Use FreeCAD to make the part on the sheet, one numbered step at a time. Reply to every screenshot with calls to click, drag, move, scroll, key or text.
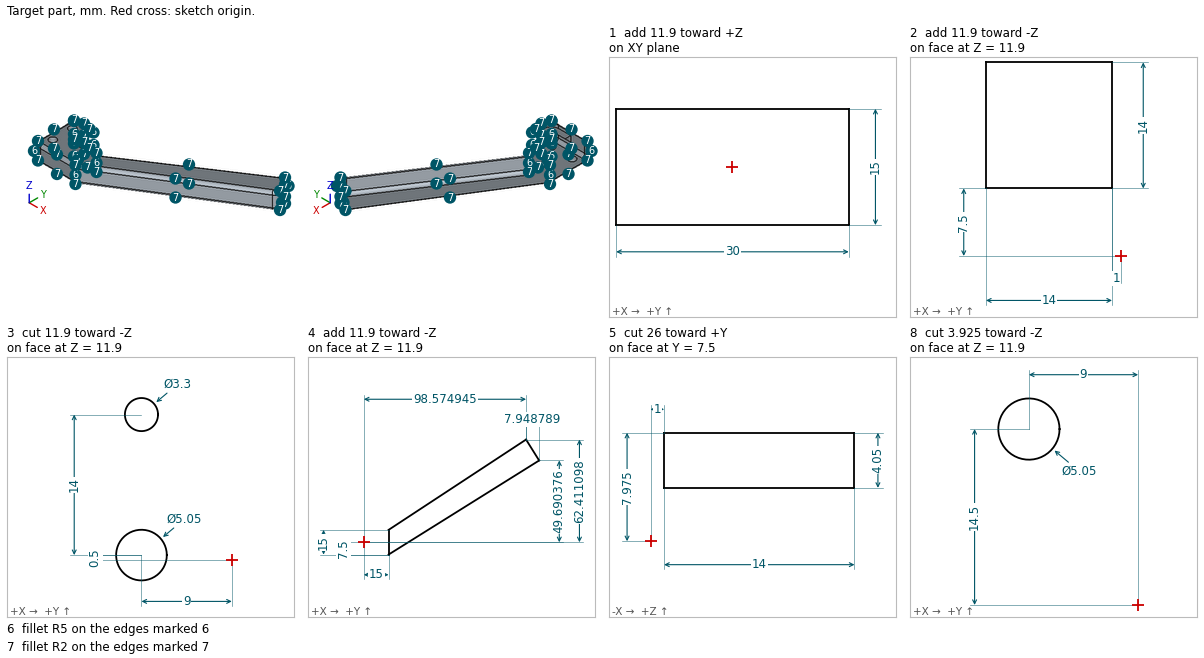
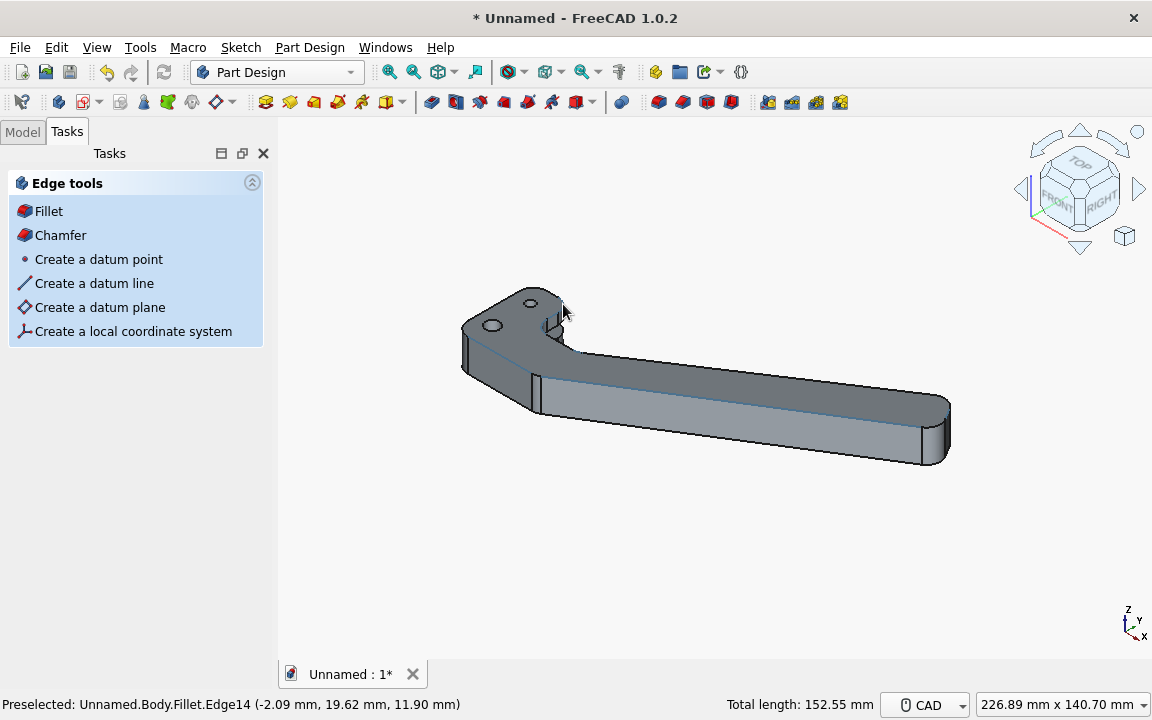
click(462, 328, ctrl)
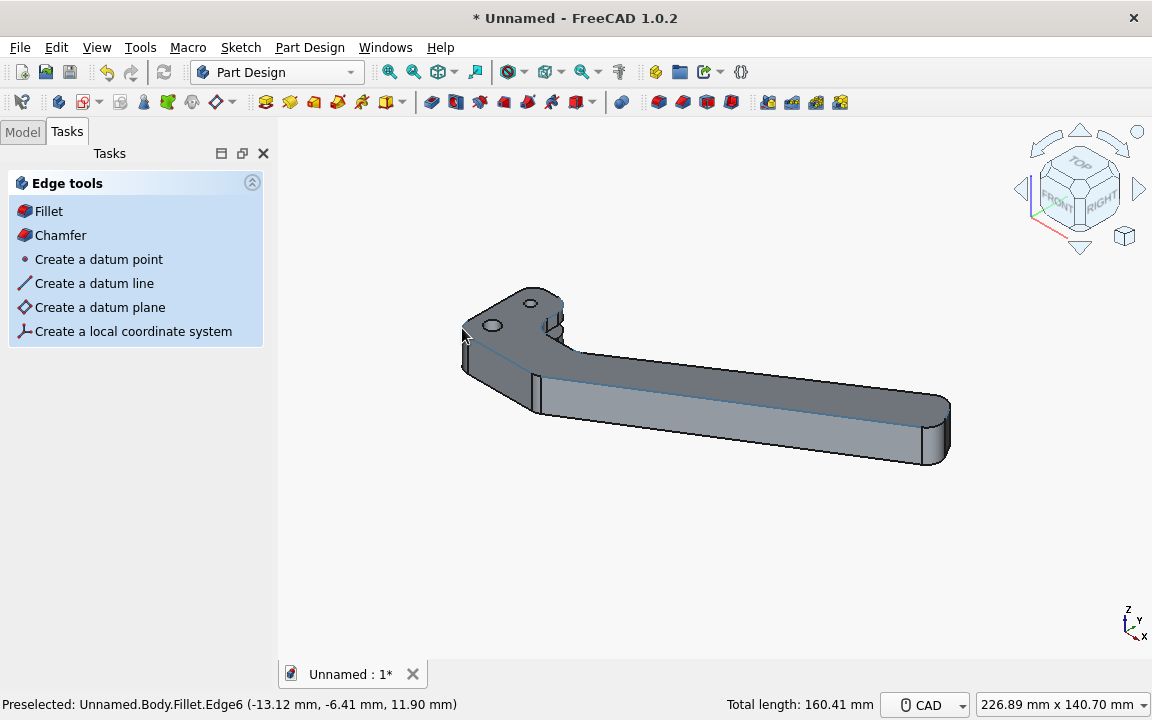
click(535, 374, ctrl)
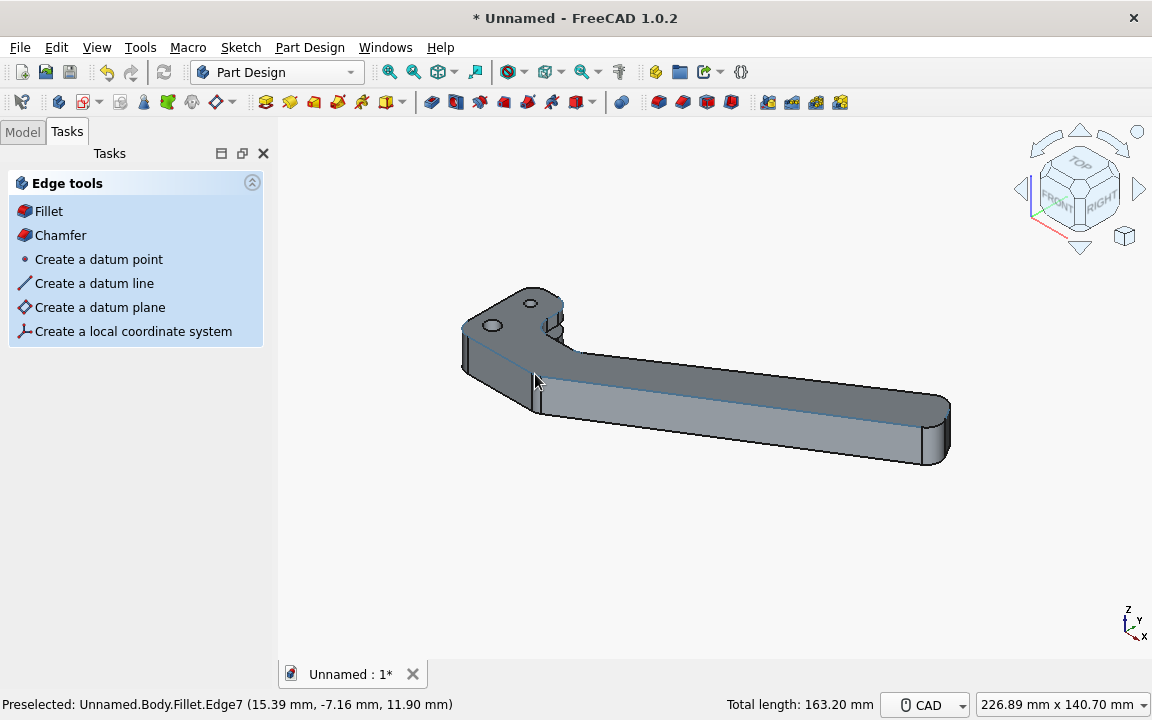
click(937, 425, ctrl)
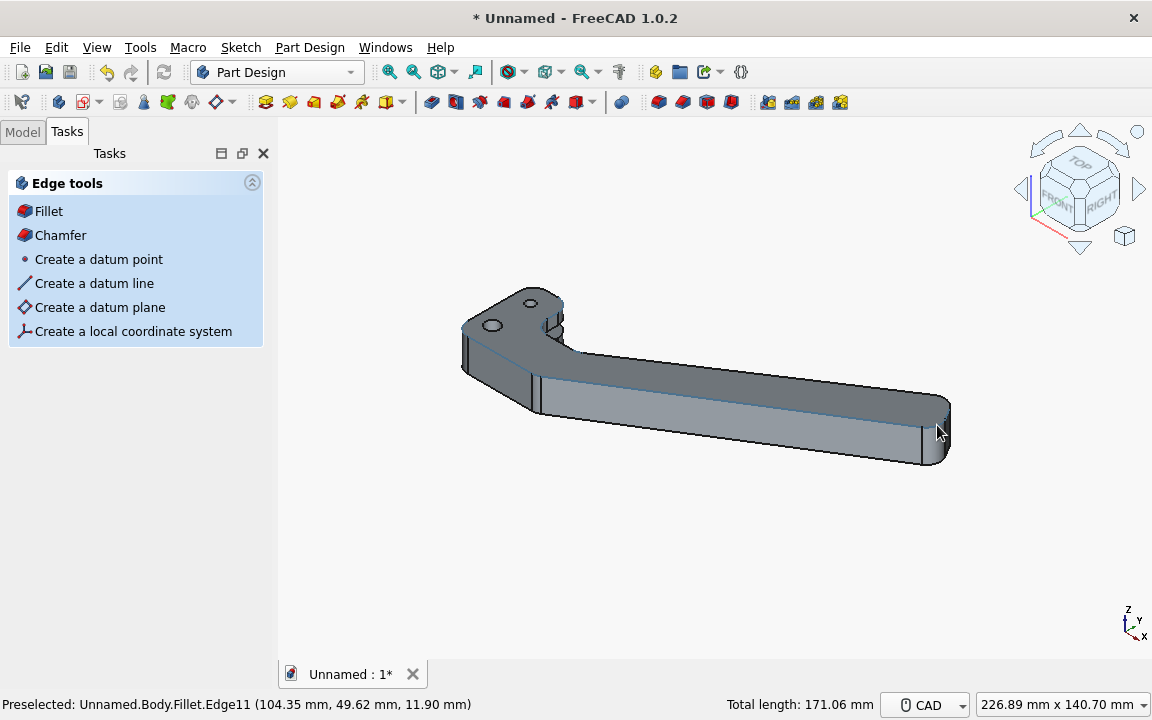
click(947, 399, ctrl)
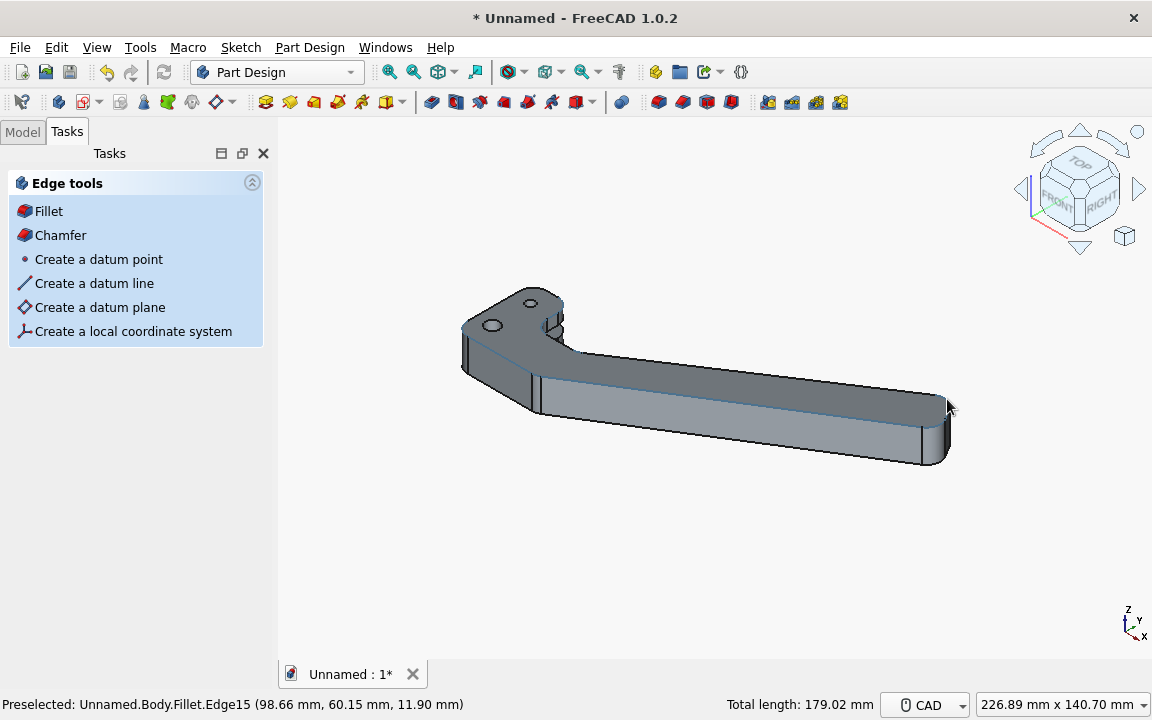
click(535, 412, ctrl)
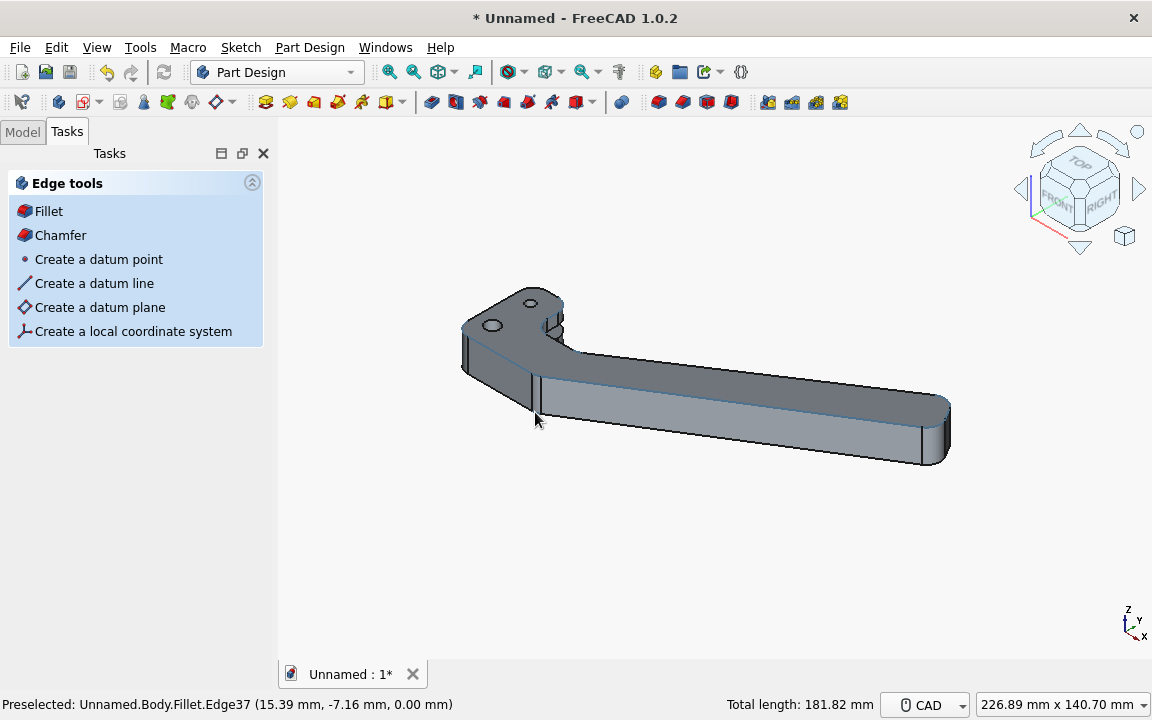
click(939, 461, ctrl)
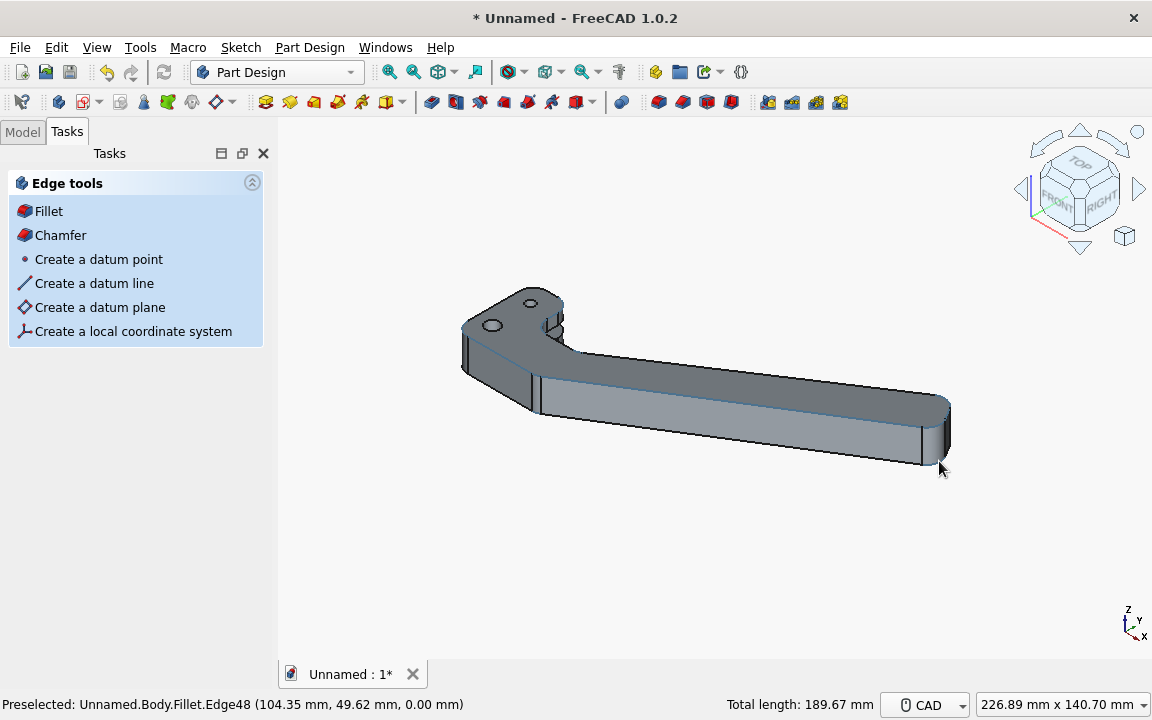
scroll(577, 388, up, 7)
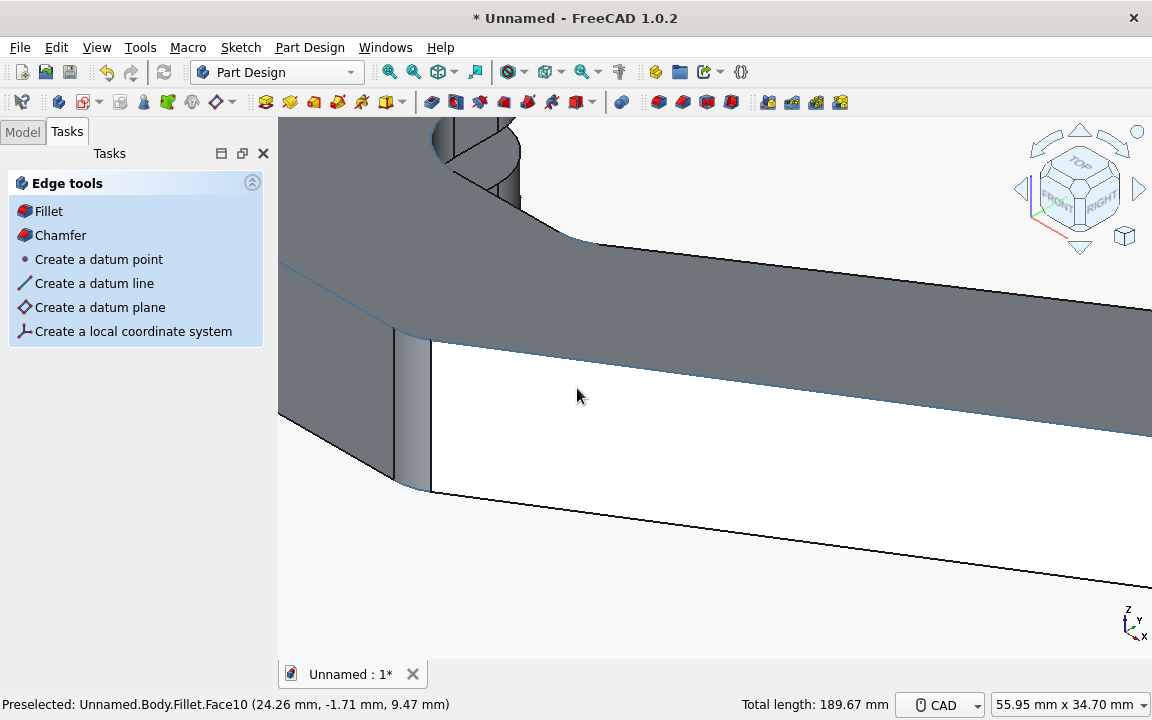
click(390, 72)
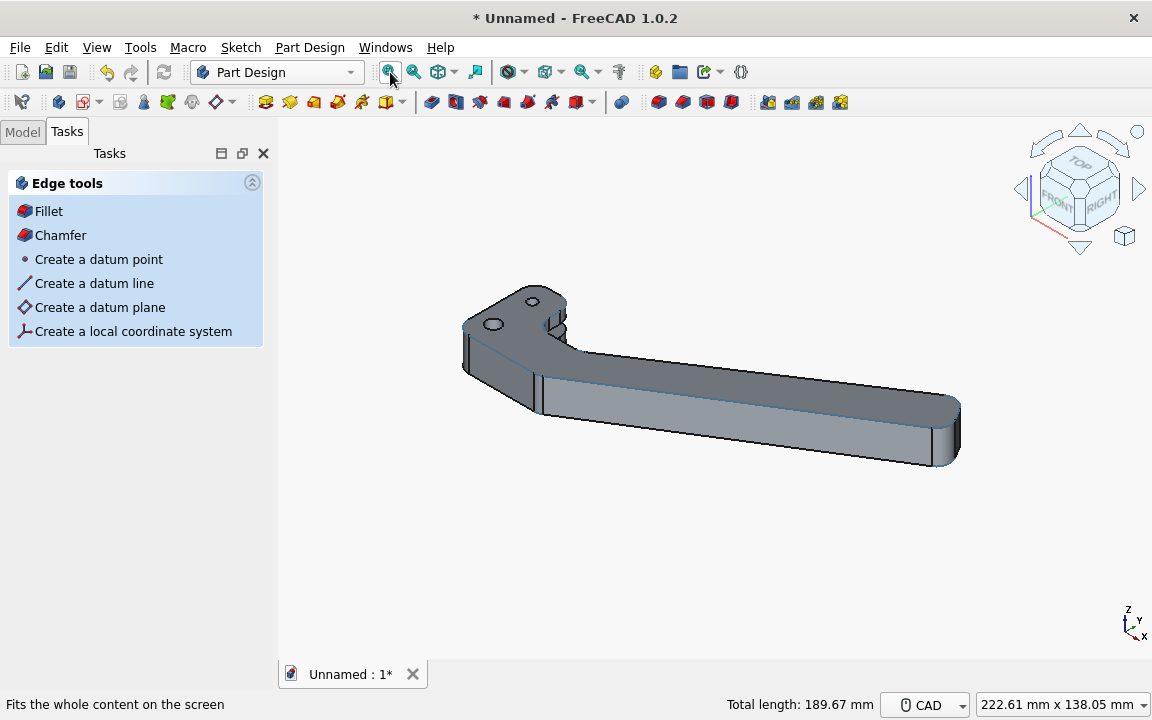
key(2)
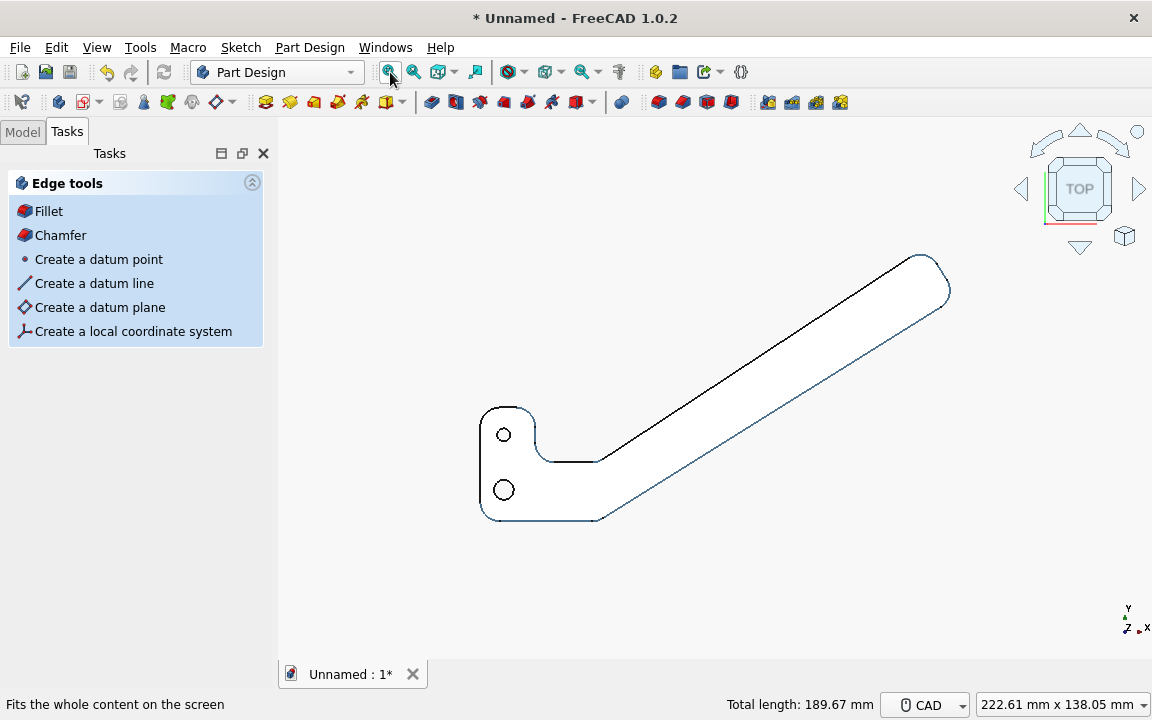
click(756, 358, ctrl)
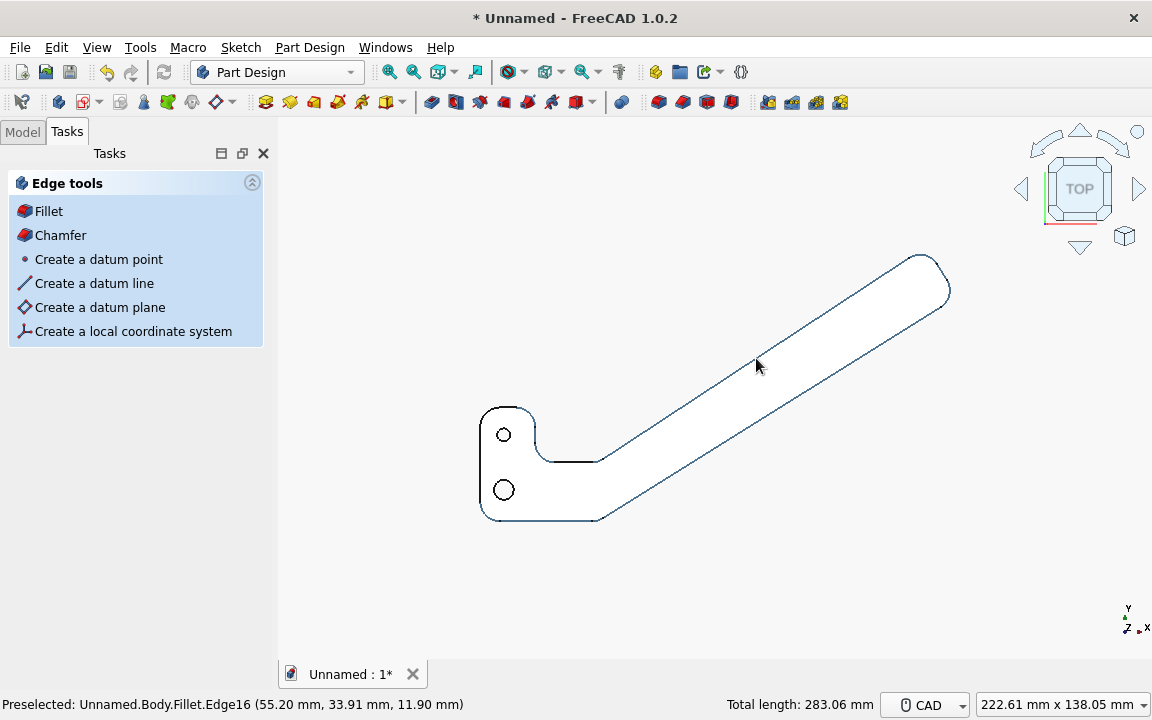
click(573, 461, ctrl)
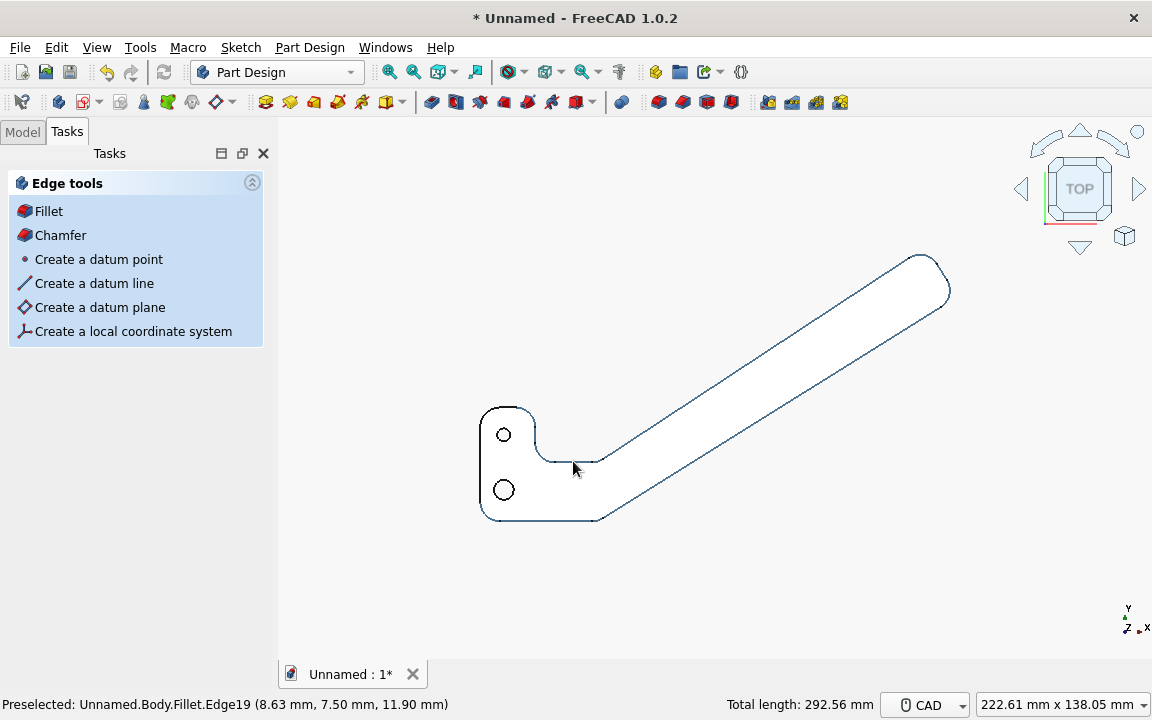
click(508, 406, ctrl)